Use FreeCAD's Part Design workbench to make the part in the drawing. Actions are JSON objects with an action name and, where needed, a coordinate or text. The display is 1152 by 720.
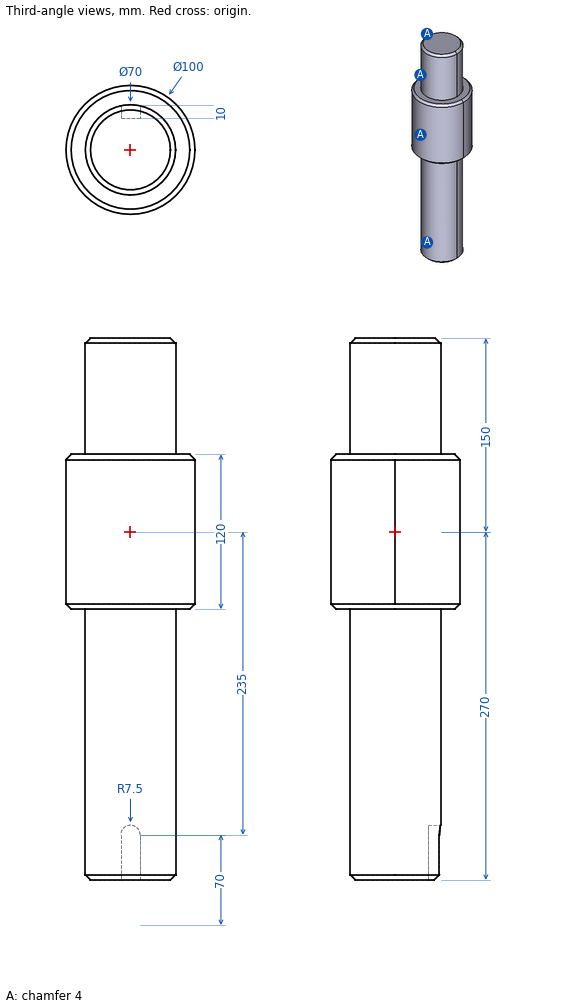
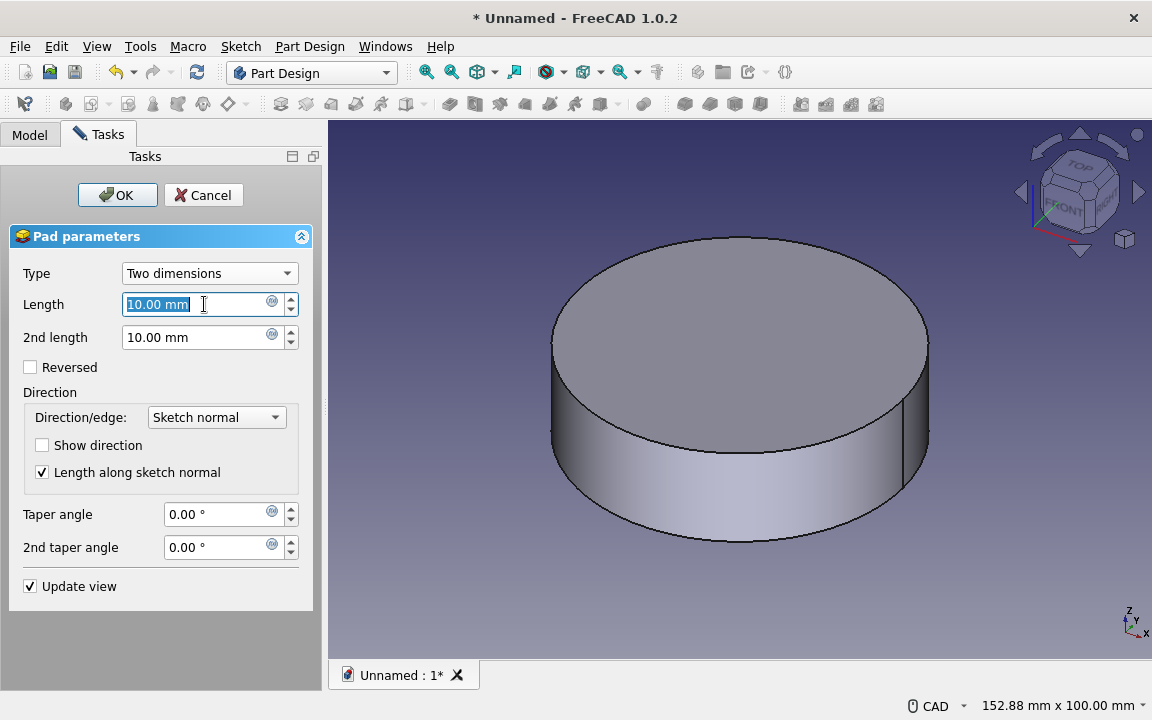
{"action": "type", "text": "150"}
{"action": "key", "text": "Tab"}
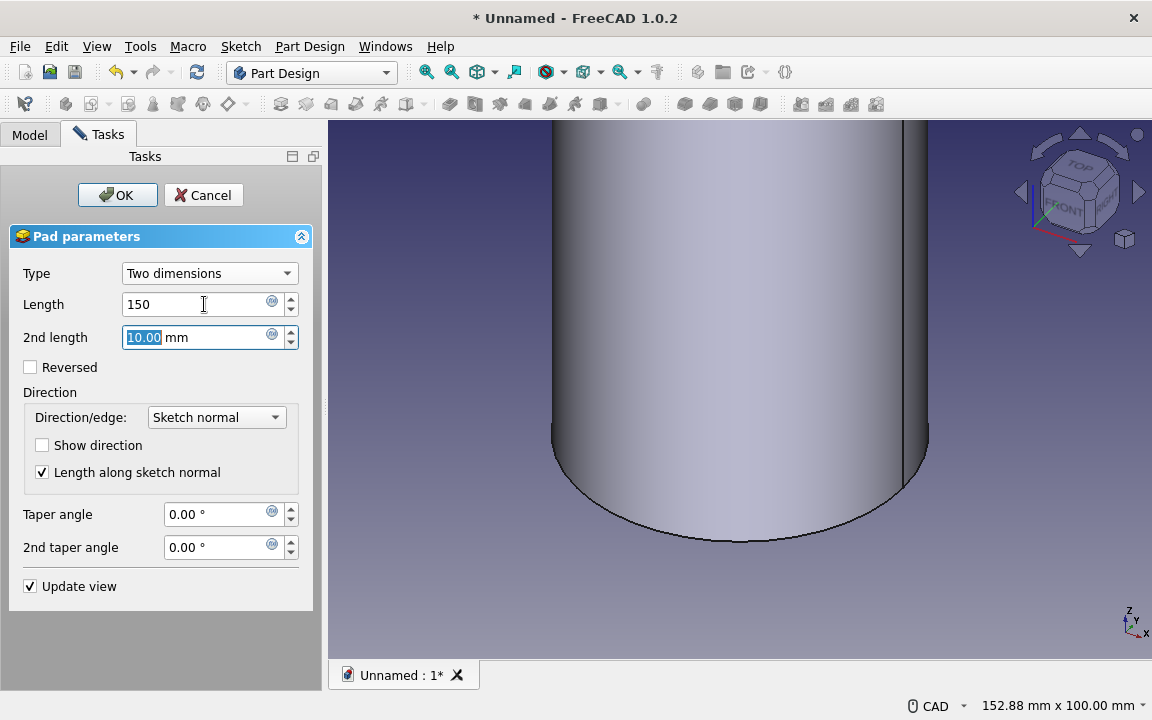
{"action": "type", "text": "270"}
{"action": "key", "text": "Tab"}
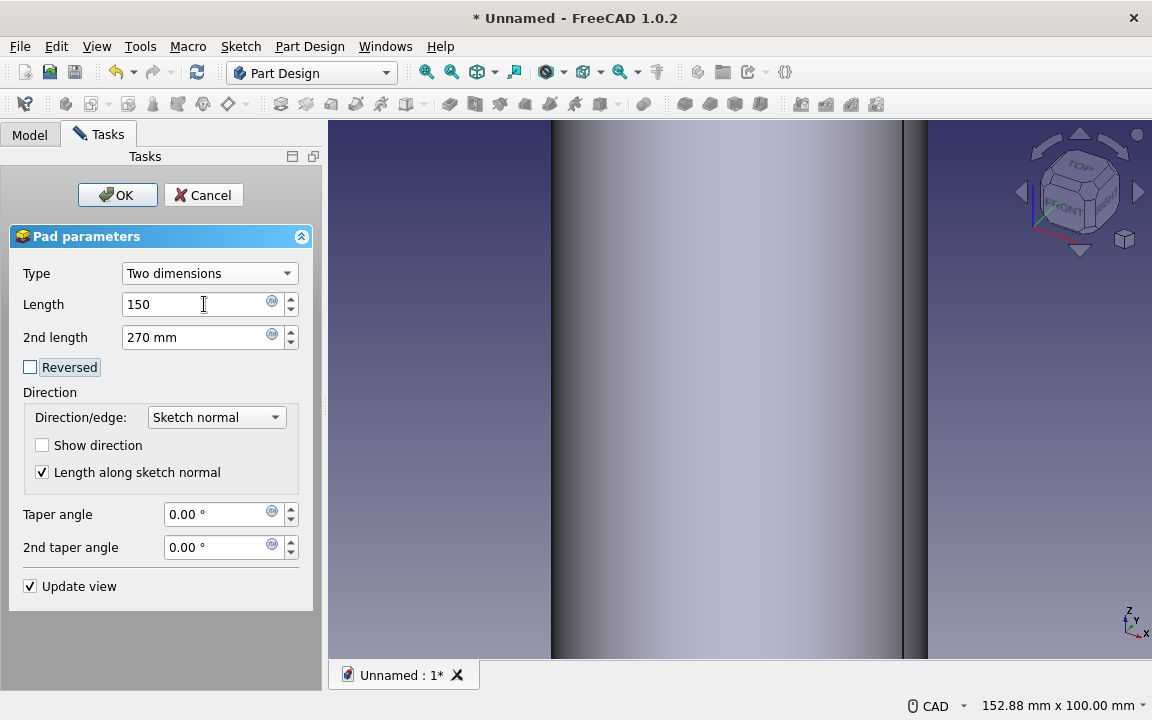
{"action": "left_click", "coordinate": [118, 195]}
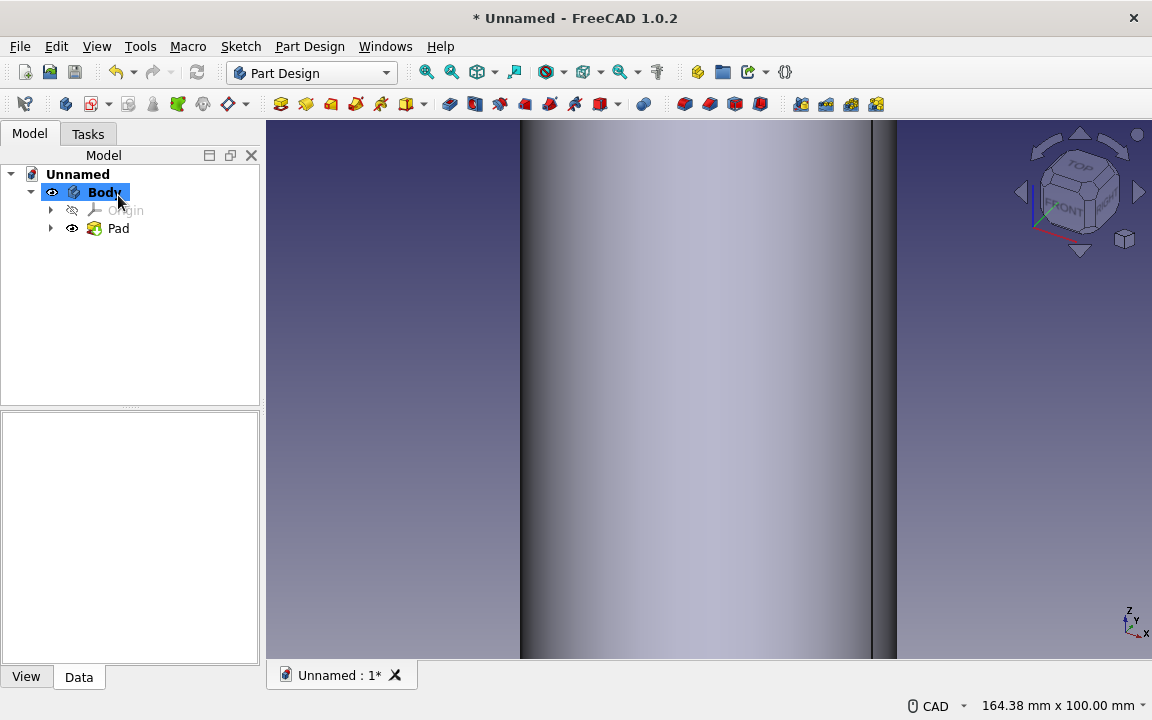
{"action": "left_click", "coordinate": [427, 72]}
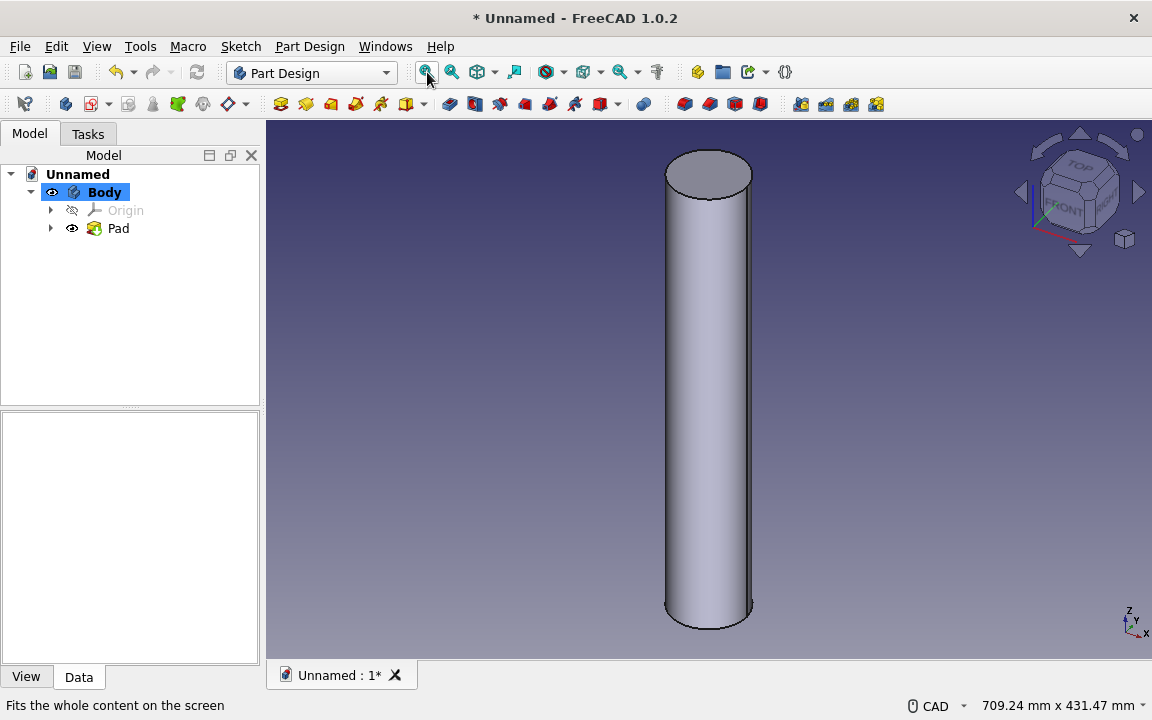
{"action": "left_click", "coordinate": [90, 104]}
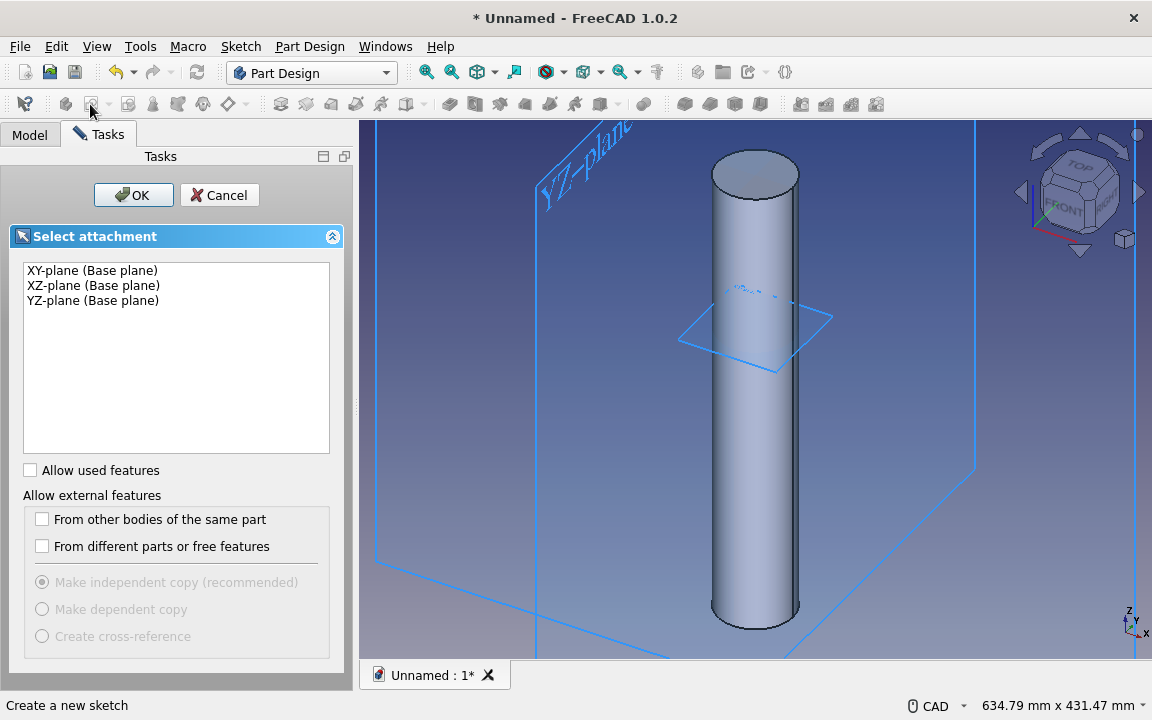
{"action": "left_click", "coordinate": [84, 270]}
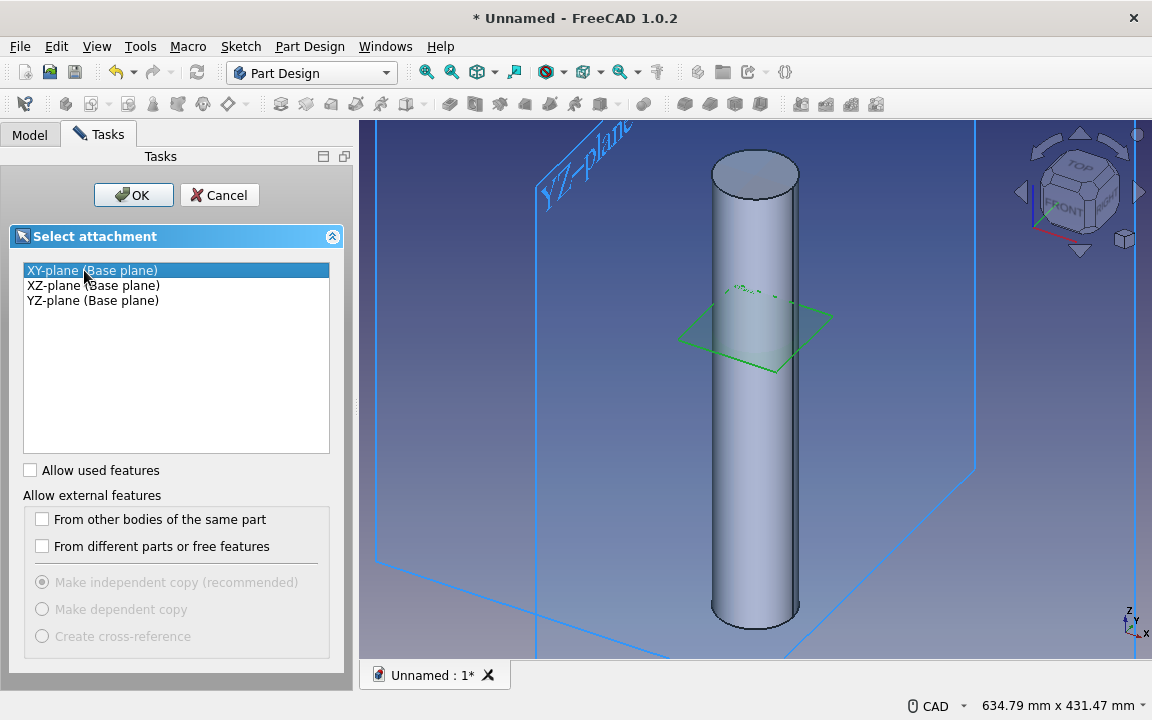
{"action": "left_click", "coordinate": [134, 195]}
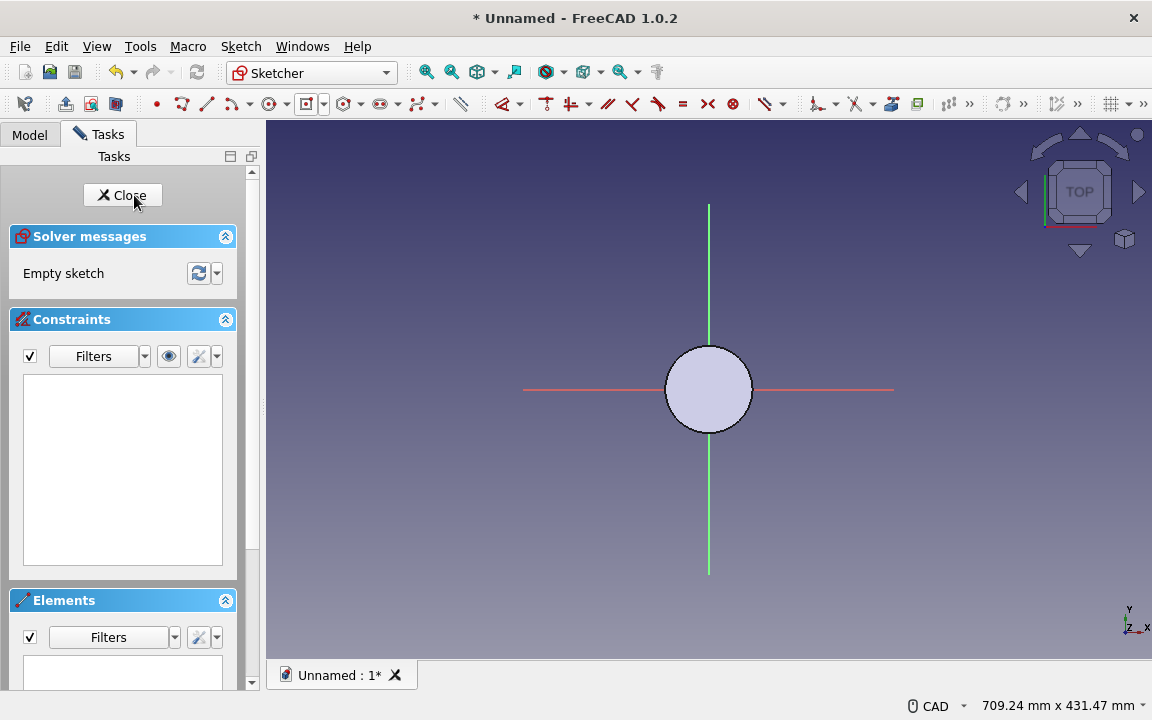
{"action": "left_click", "coordinate": [116, 104]}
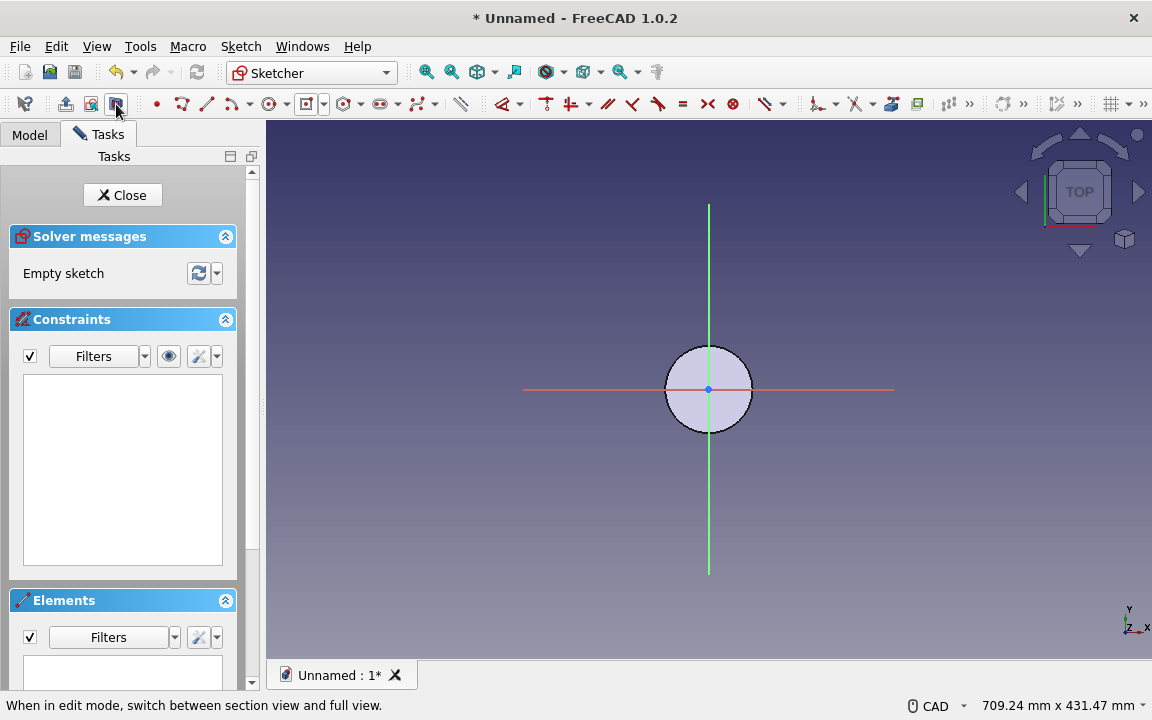
{"action": "scroll", "coordinate": [749, 390], "scroll_direction": "up", "scroll_amount": 5}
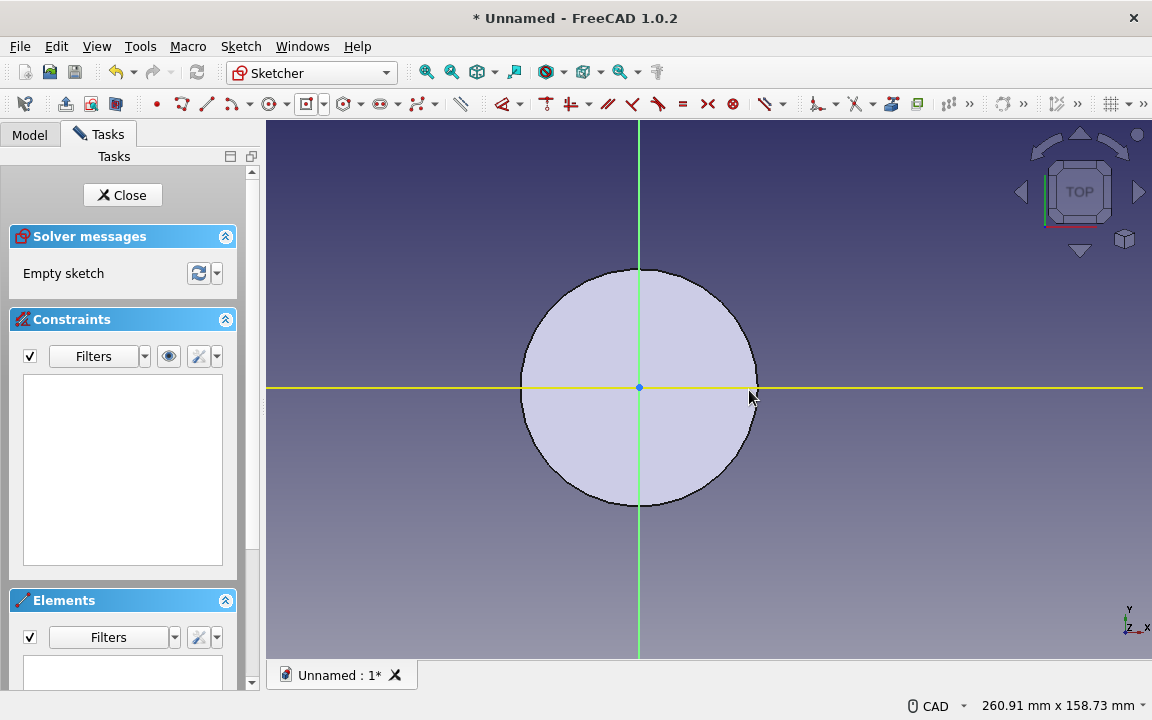
{"action": "key", "text": "g c"}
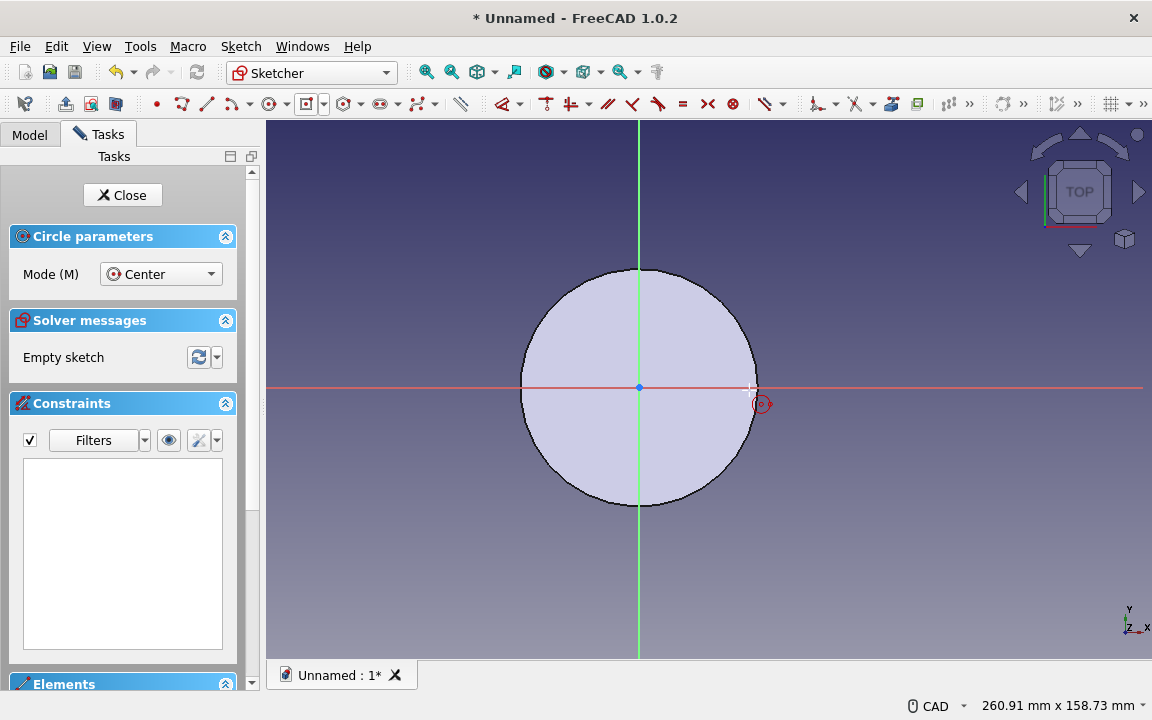
{"action": "left_click", "coordinate": [639, 388]}
{"action": "mouse_move", "coordinate": [759, 268]}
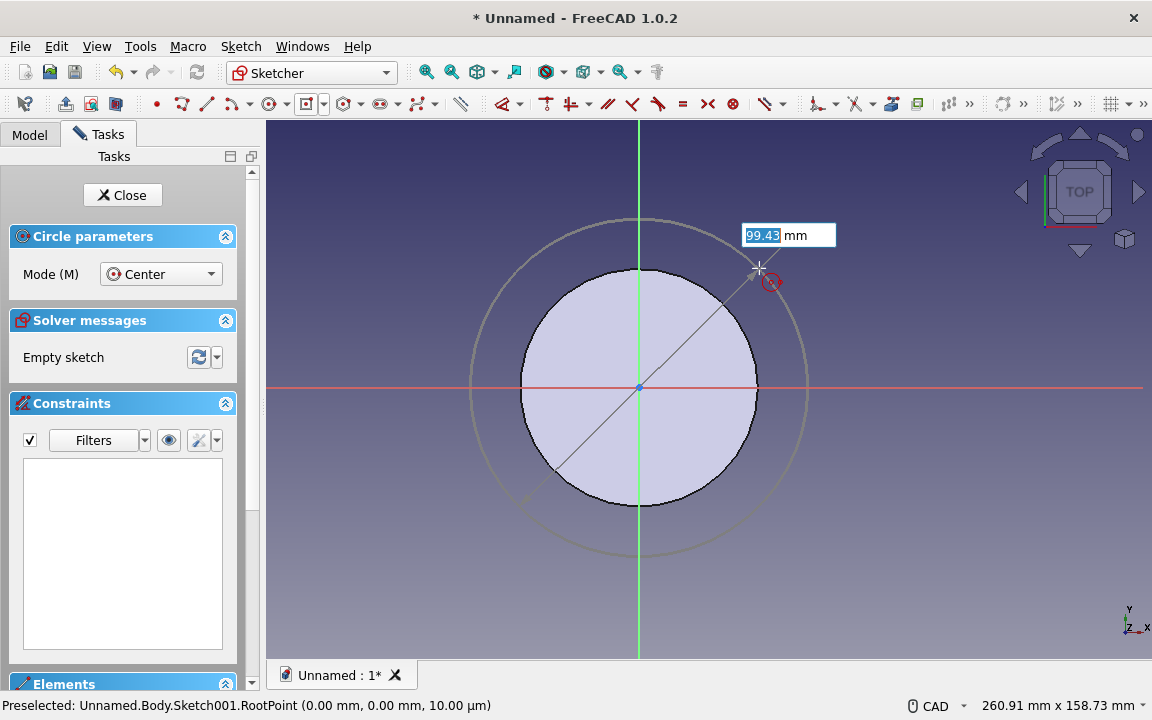
{"action": "type", "text": "100"}
{"action": "key", "text": "Return"}
{"action": "key", "text": "Escape"}